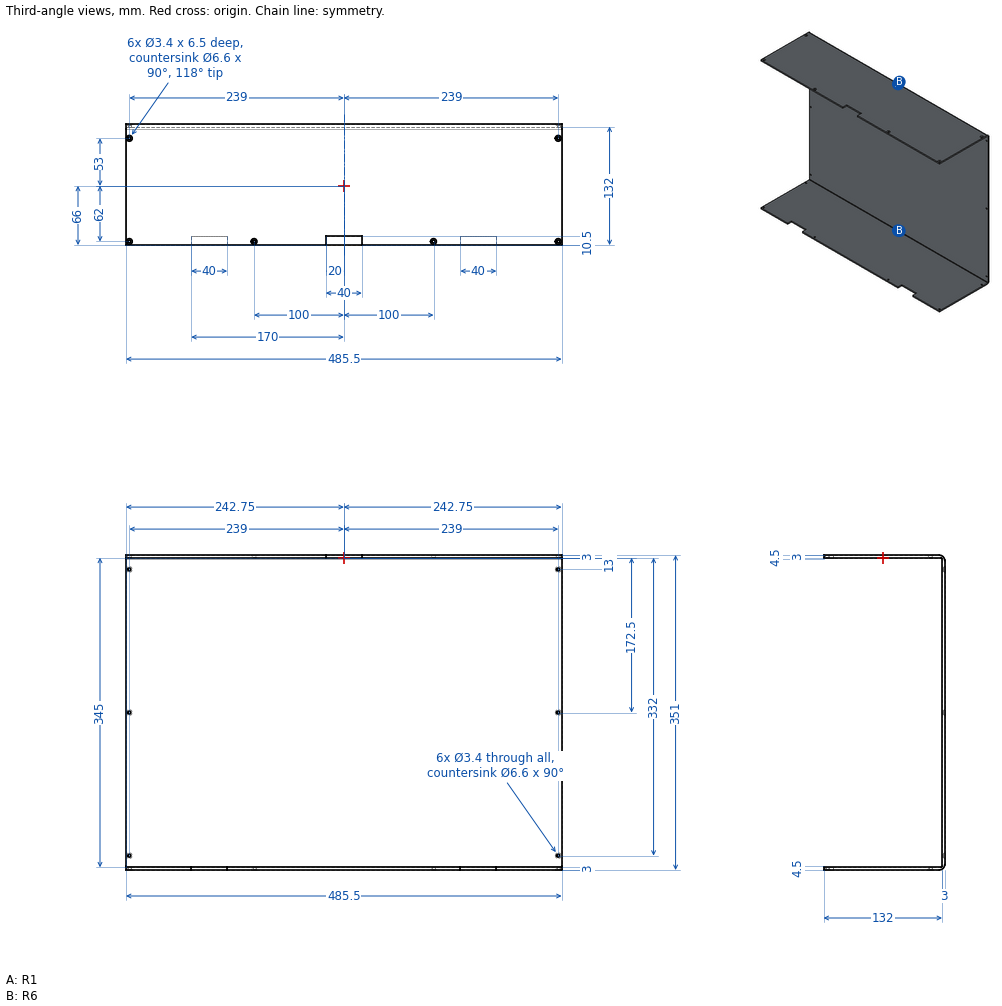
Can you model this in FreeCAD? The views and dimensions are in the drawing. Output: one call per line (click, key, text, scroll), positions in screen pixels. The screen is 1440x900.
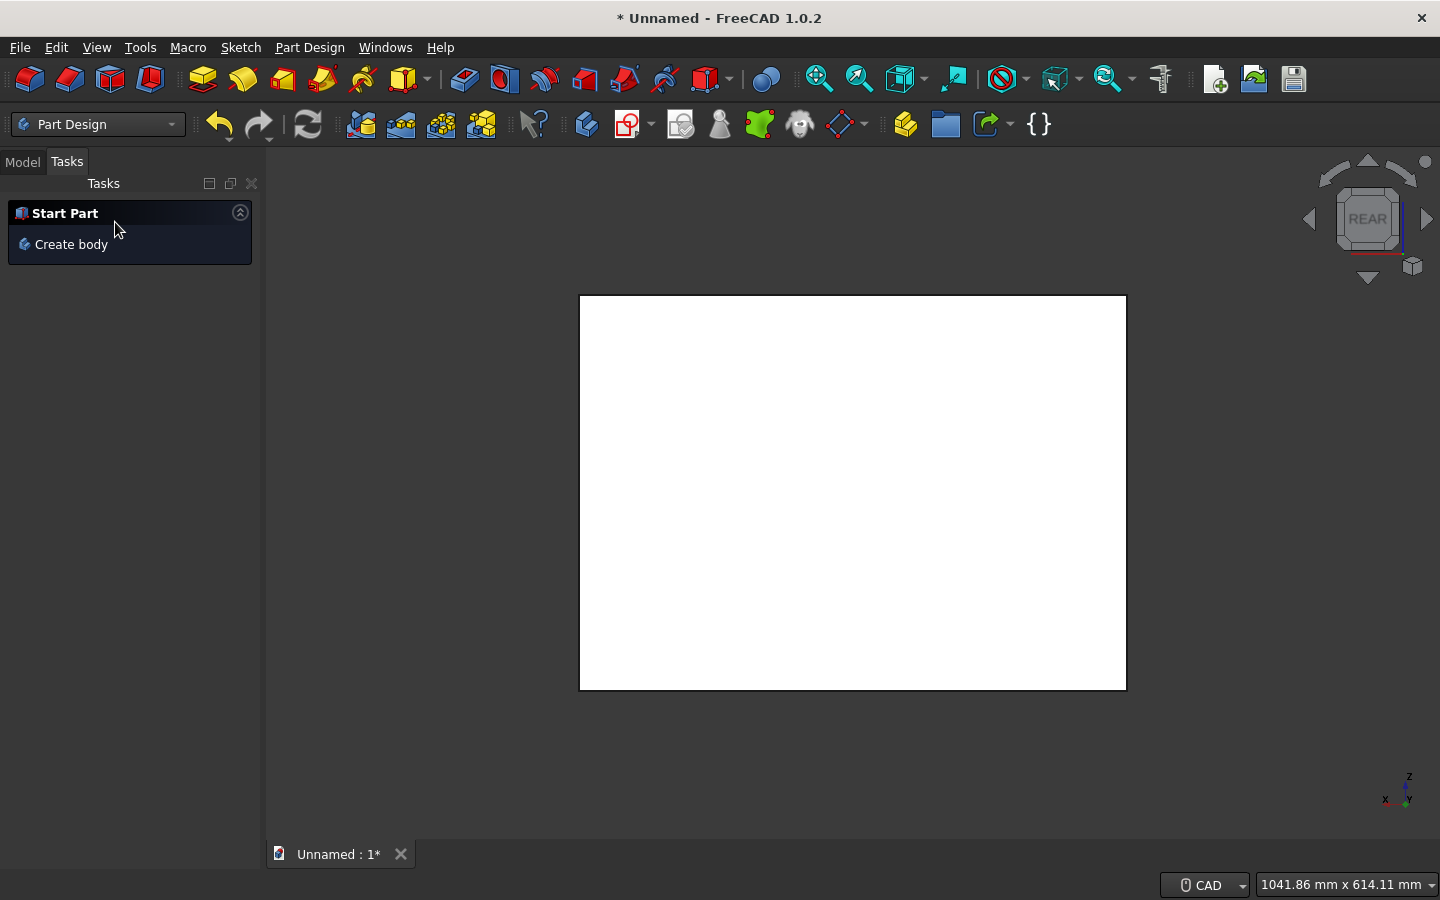
key(6)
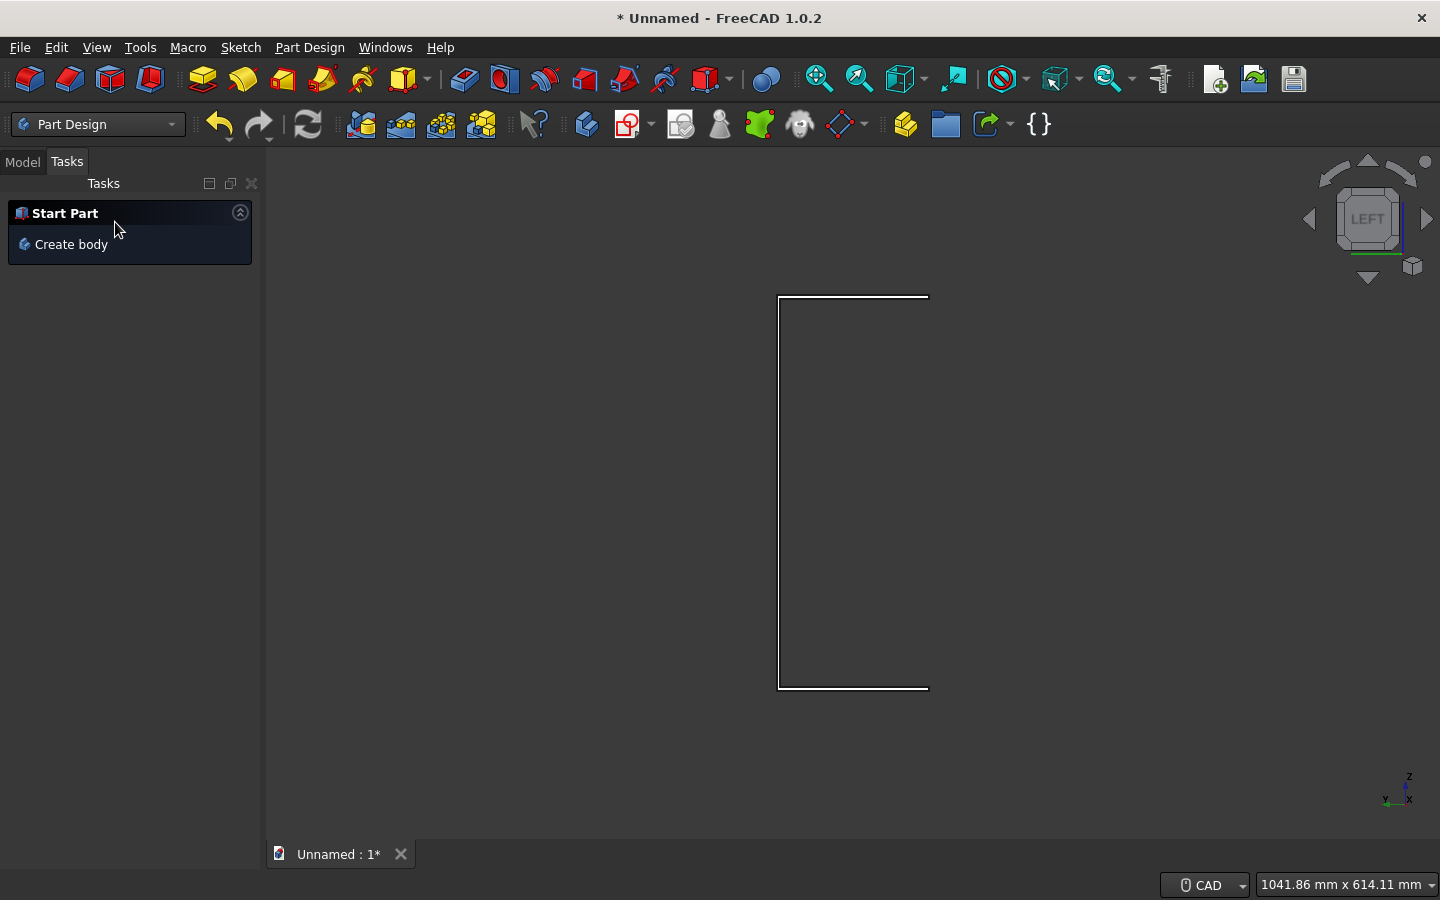
key(v)
key(3)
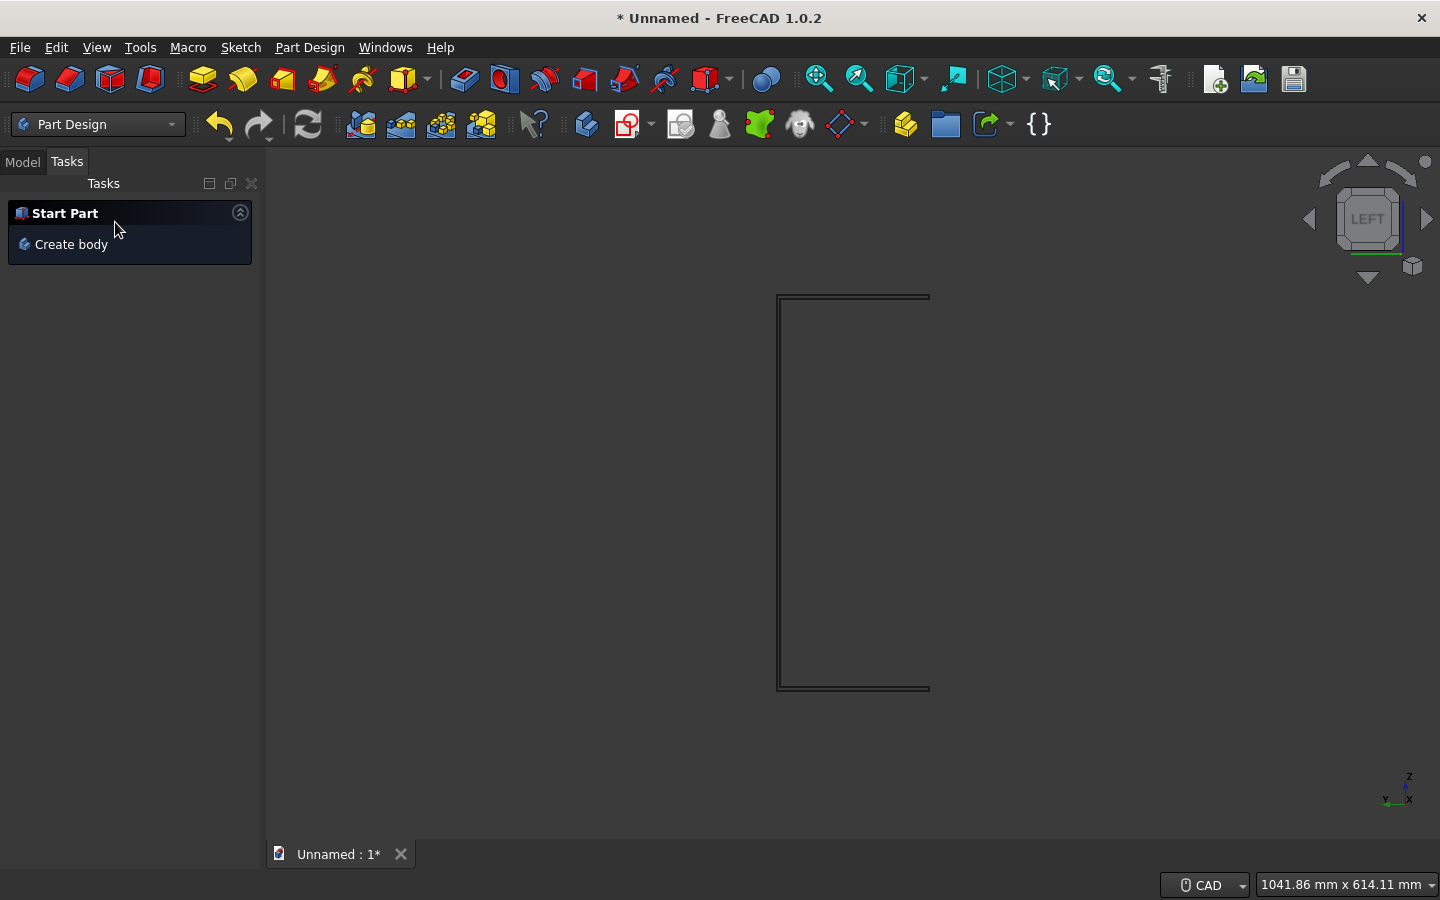
key(0)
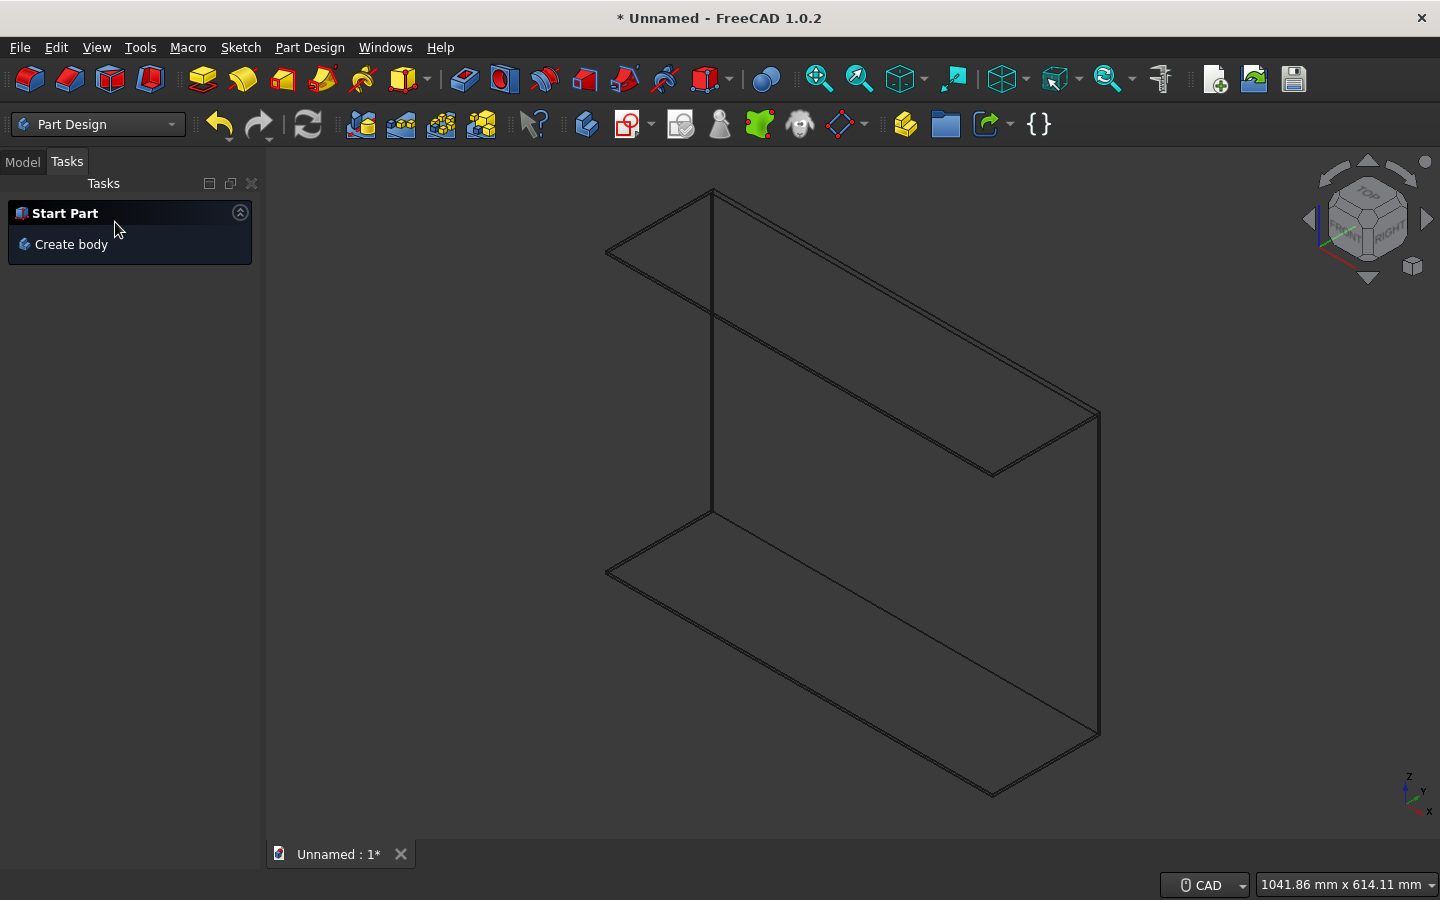
click(904, 621)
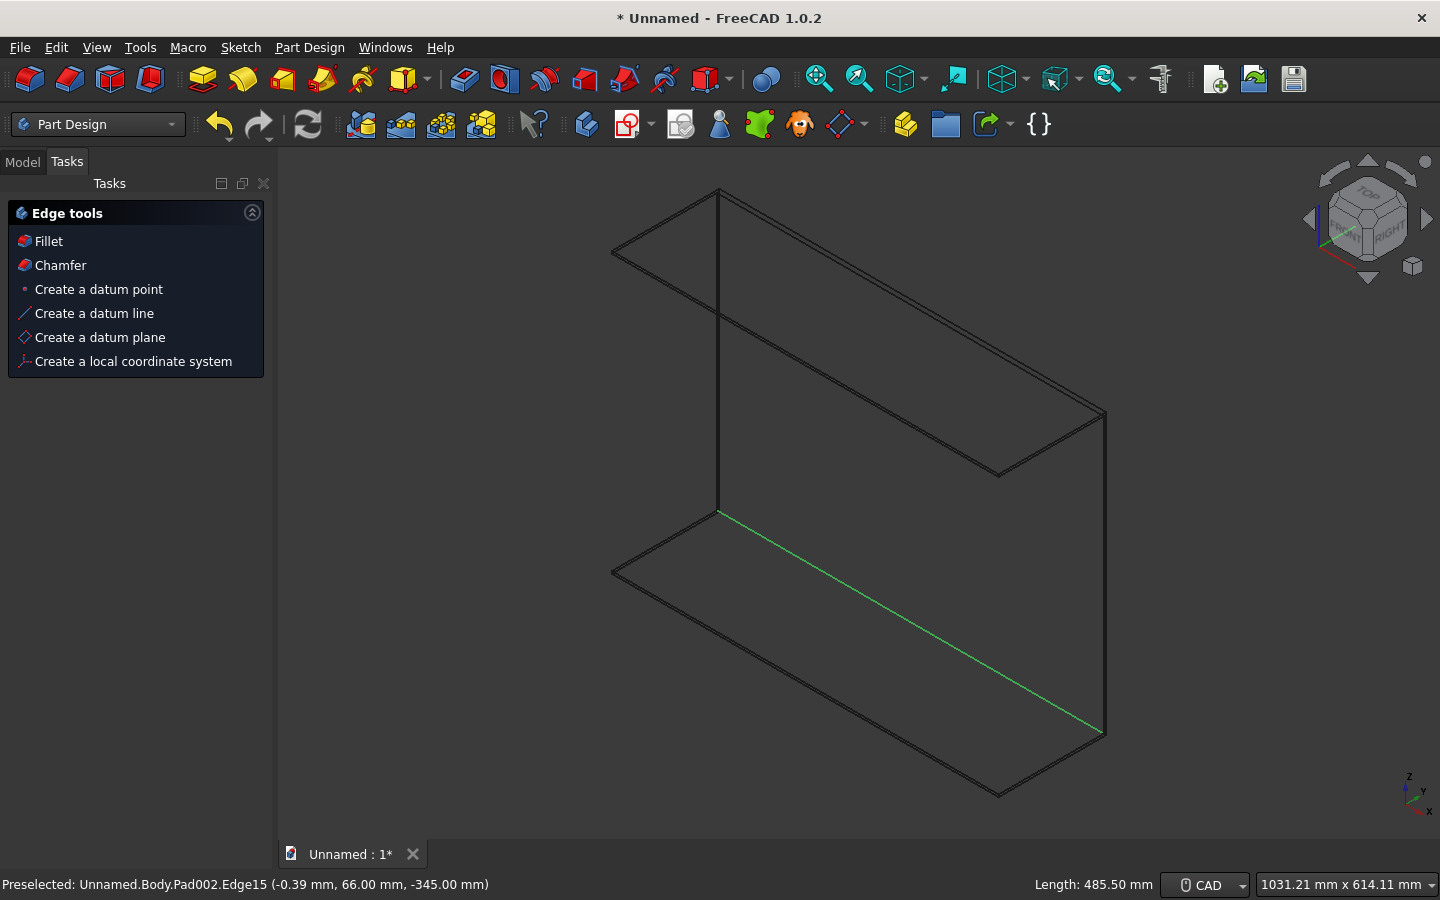
scroll(910, 304, up, 6)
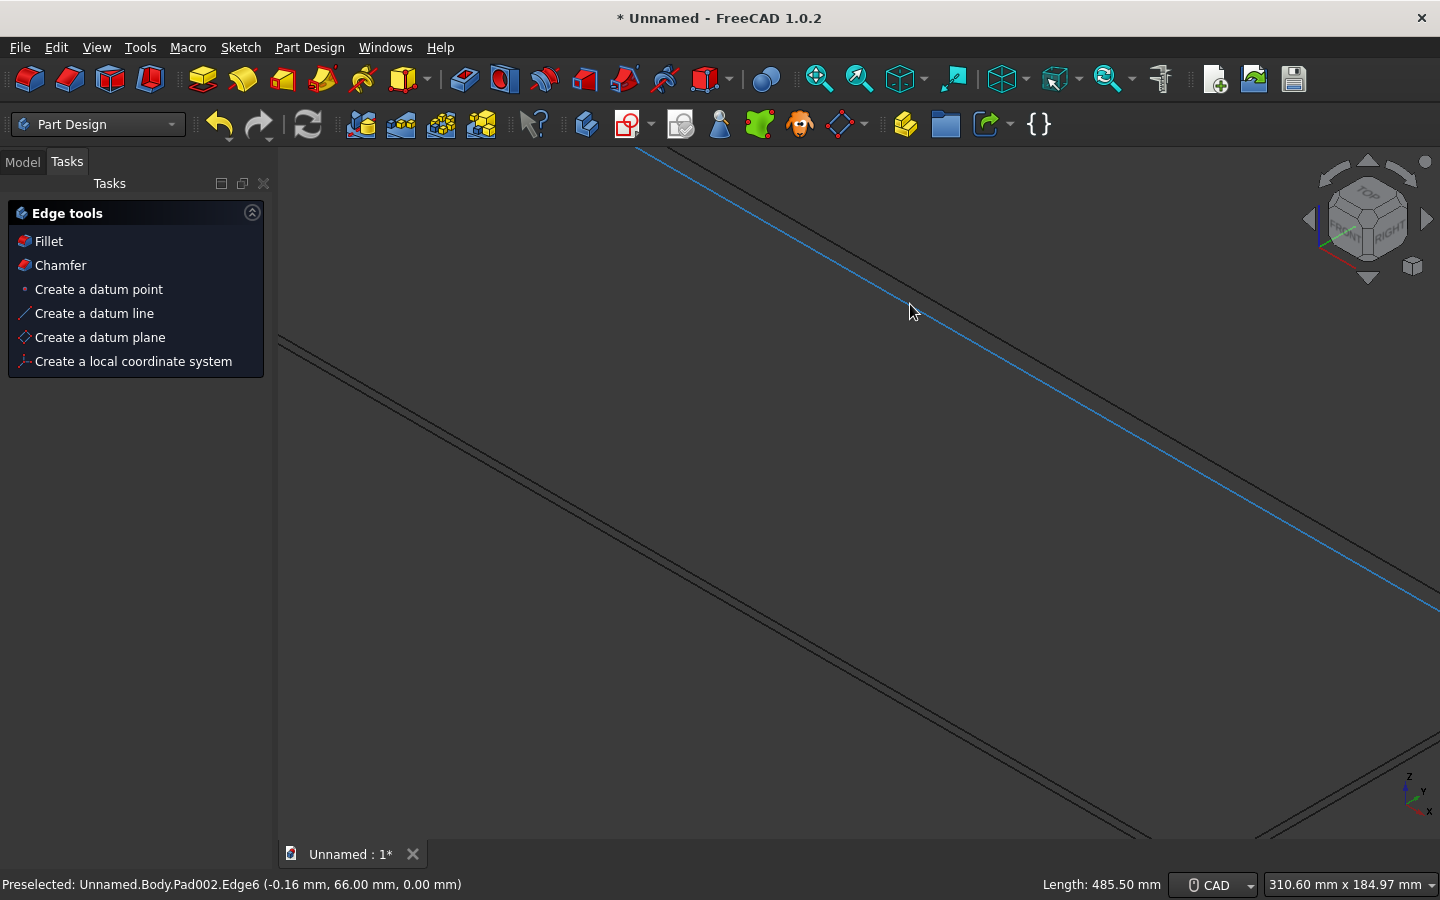
click(910, 305, ctrl)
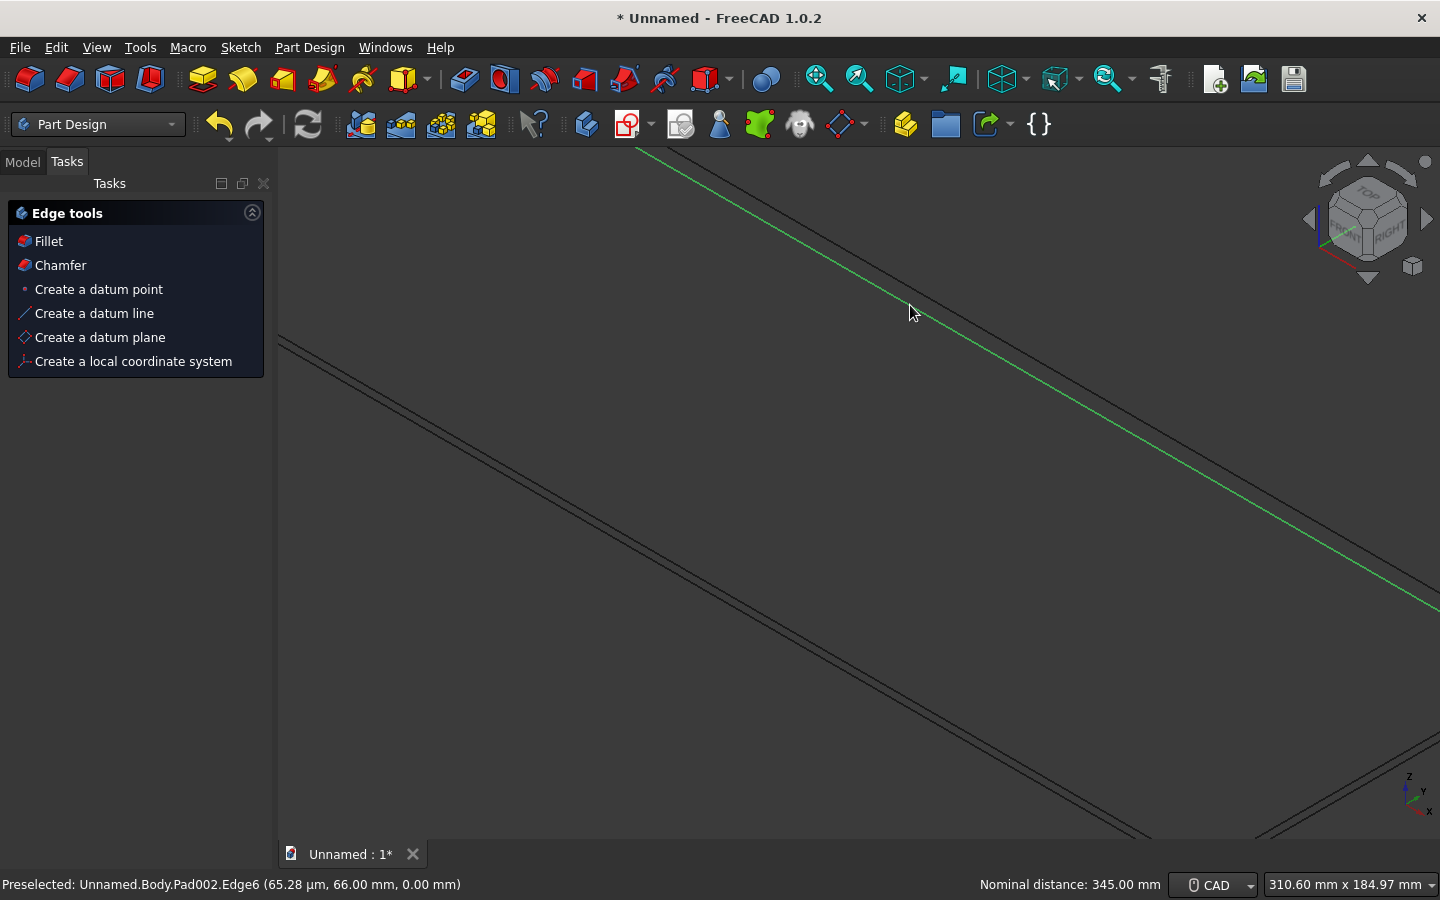
key(v)
key(1)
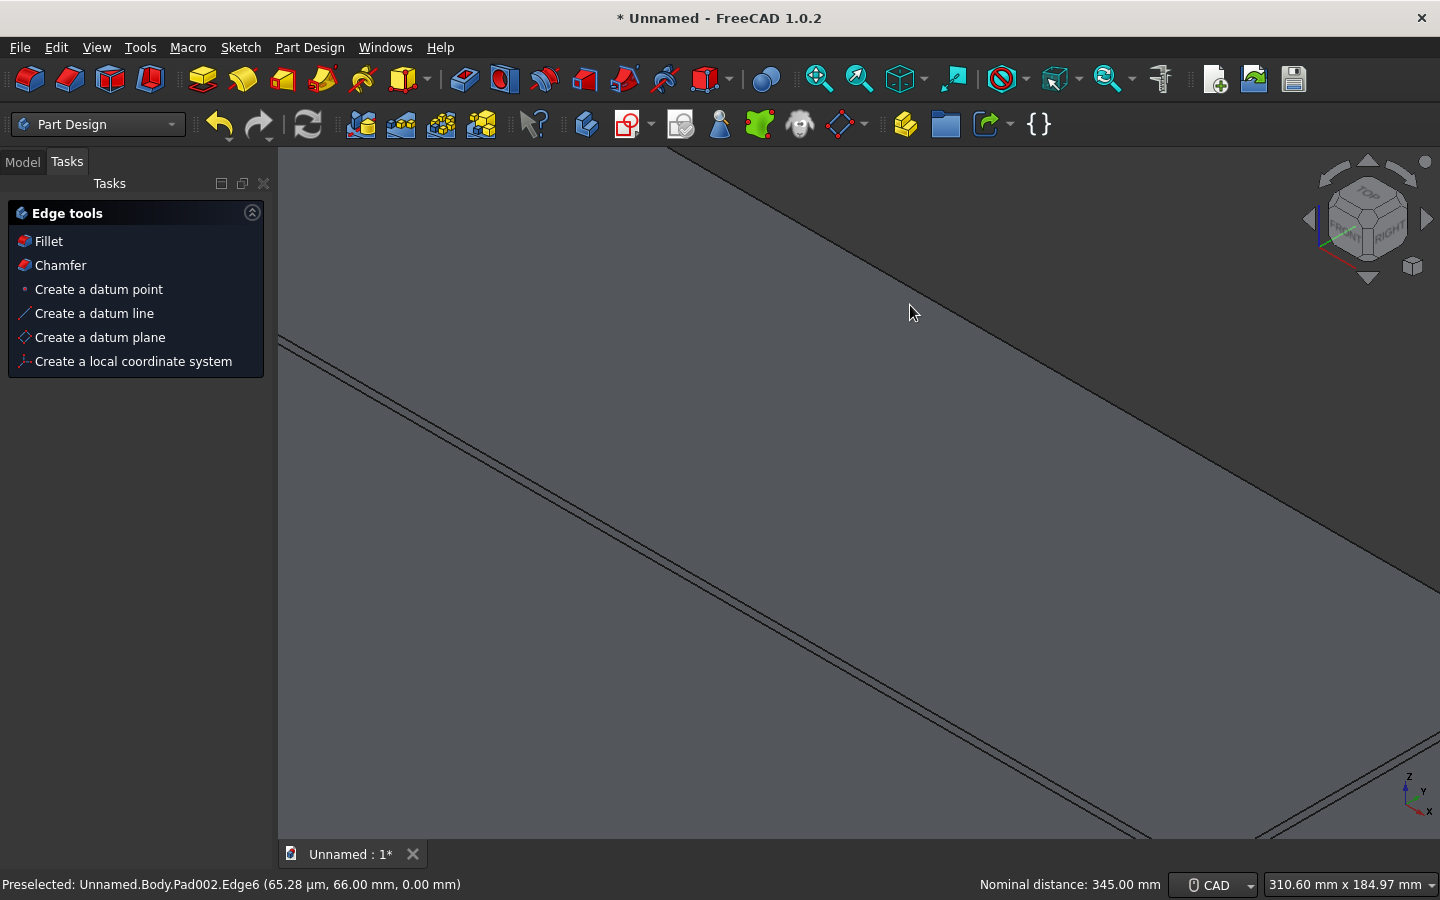
click(30, 80)